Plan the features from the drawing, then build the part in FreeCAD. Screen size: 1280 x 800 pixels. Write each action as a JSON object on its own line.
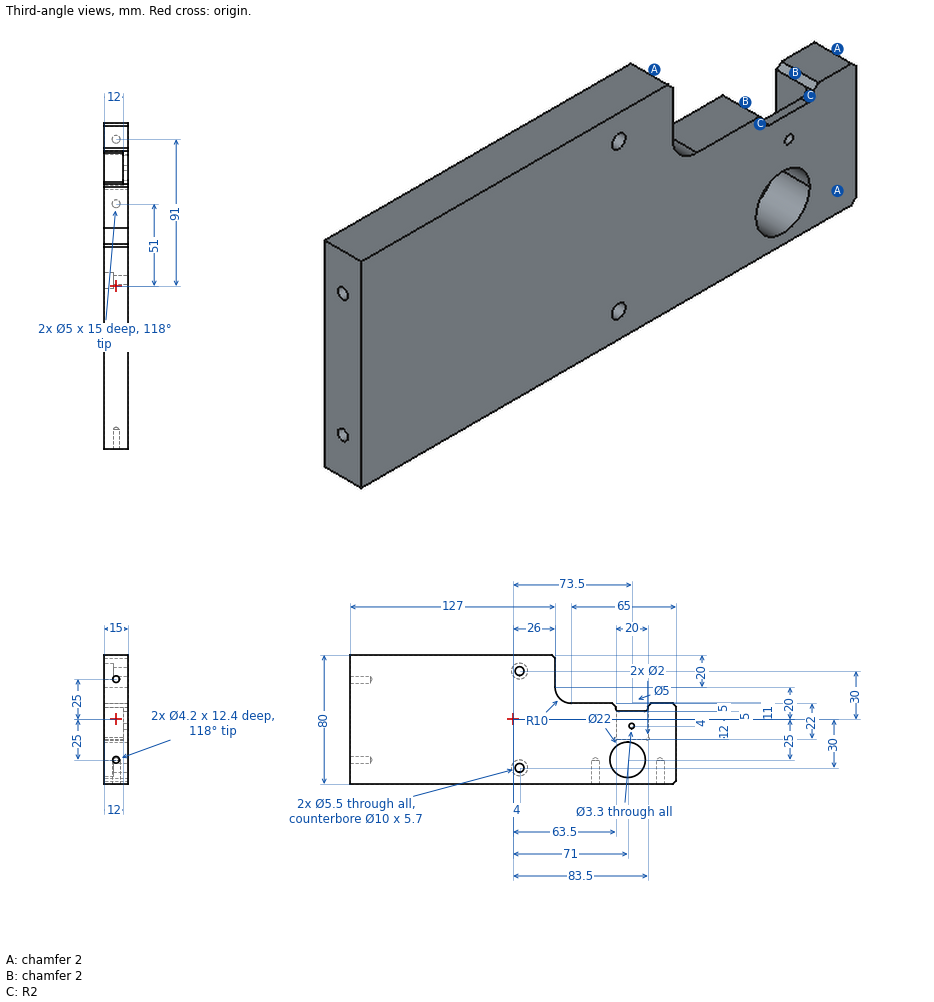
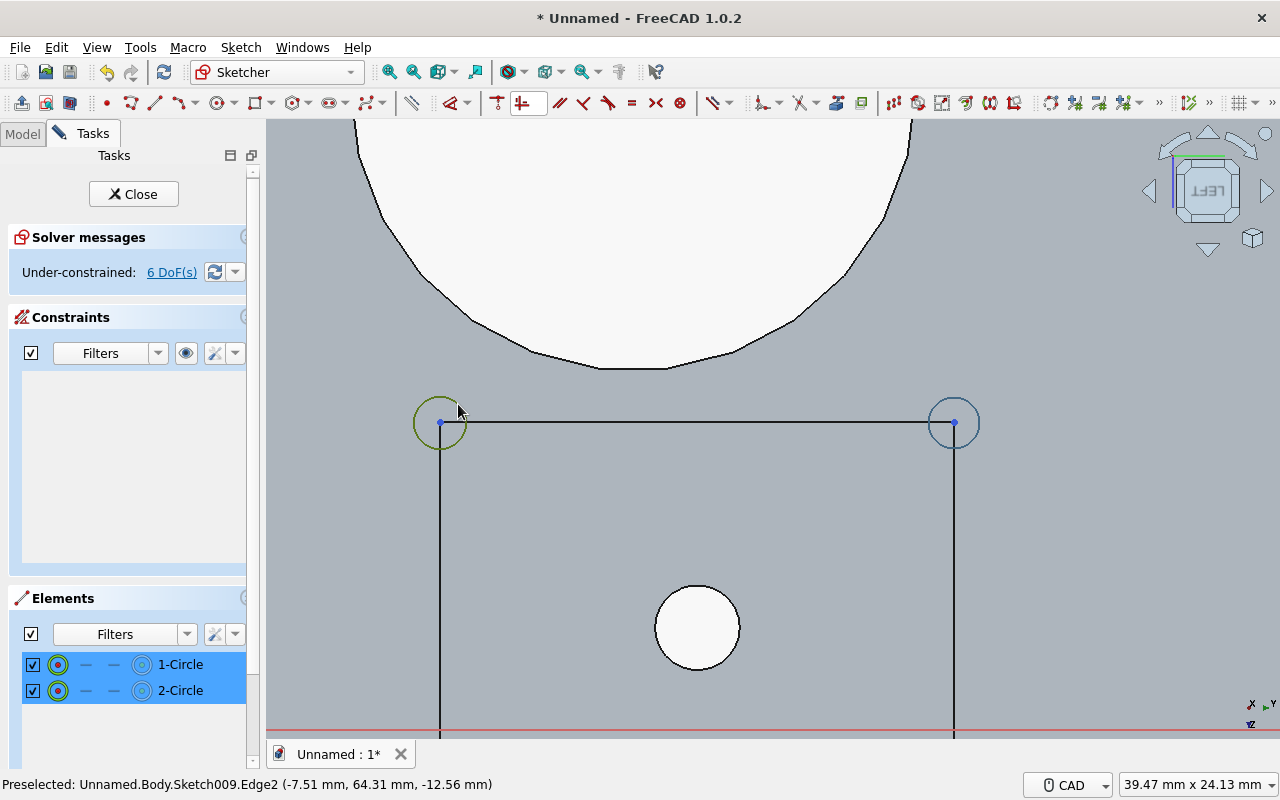
{"action": "left_click", "coordinate": [632, 104]}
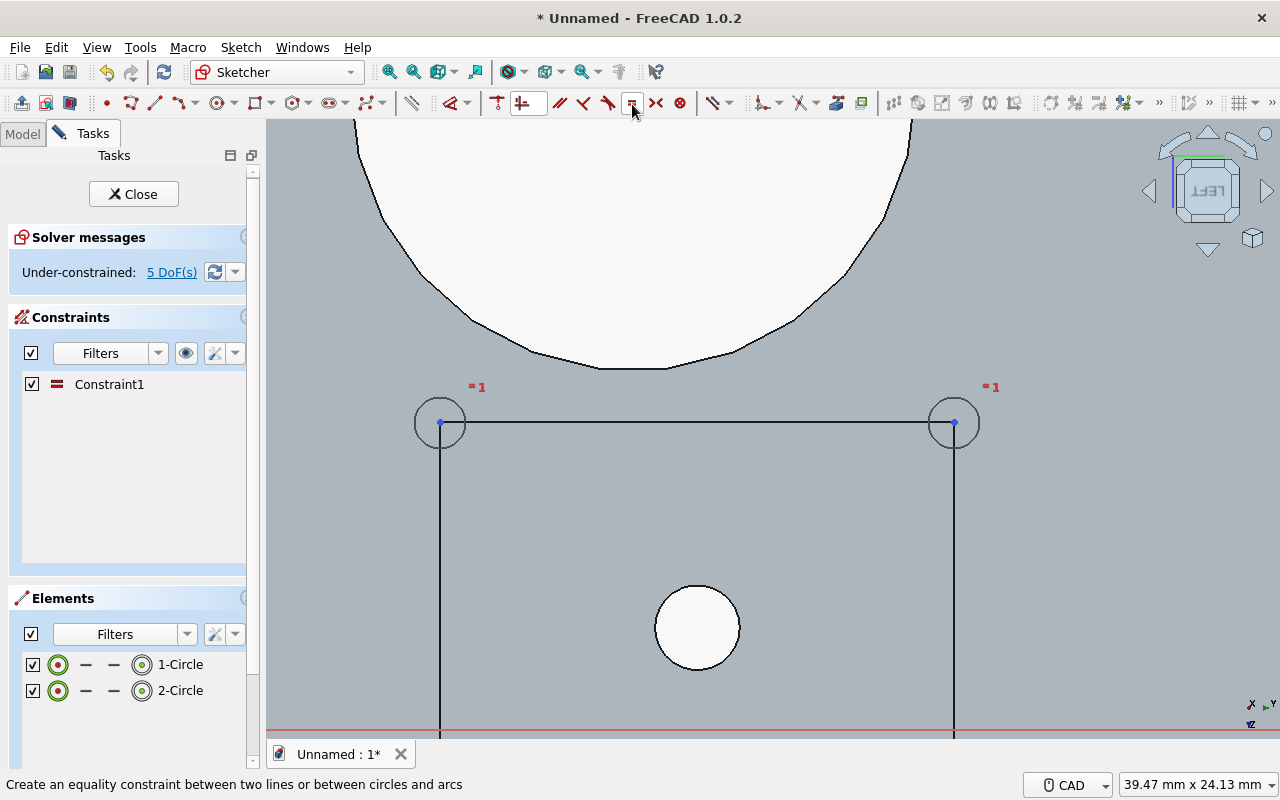
{"action": "left_click", "coordinate": [954, 423]}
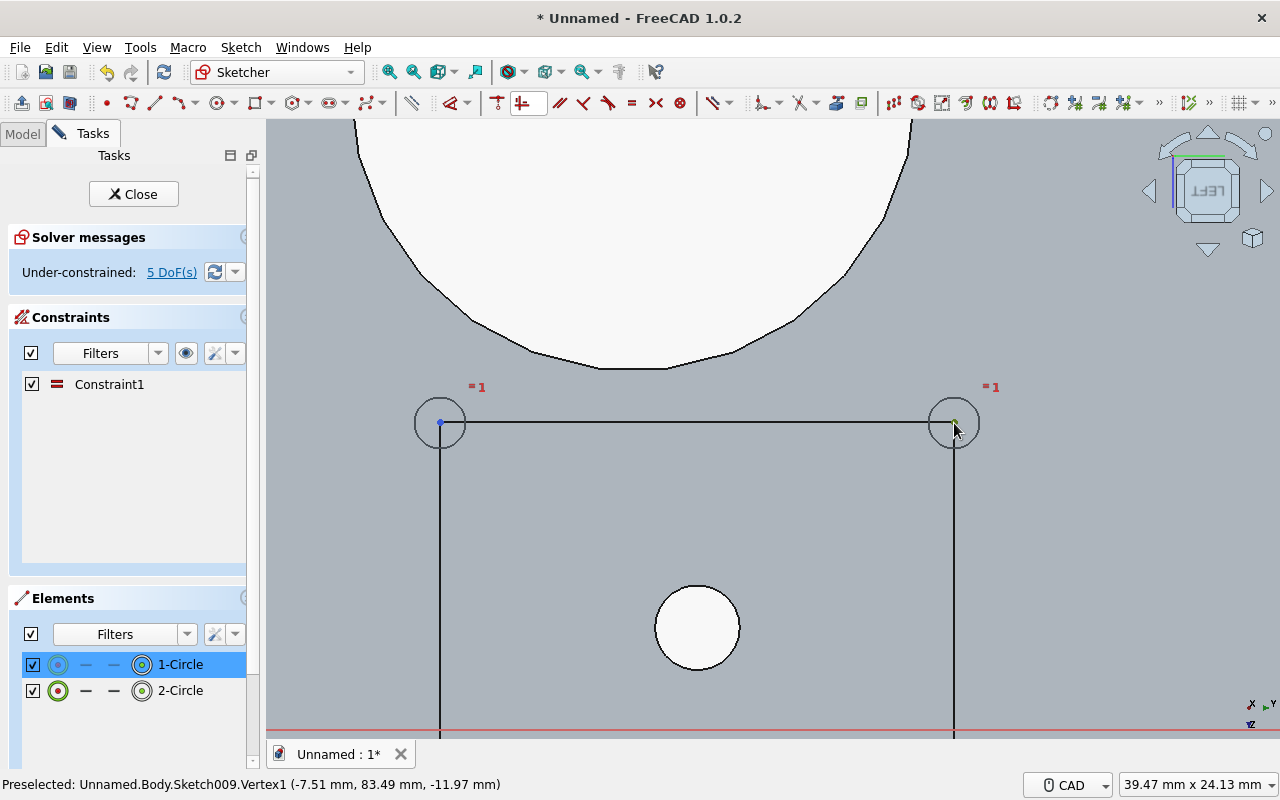
{"action": "left_click", "coordinate": [440, 423]}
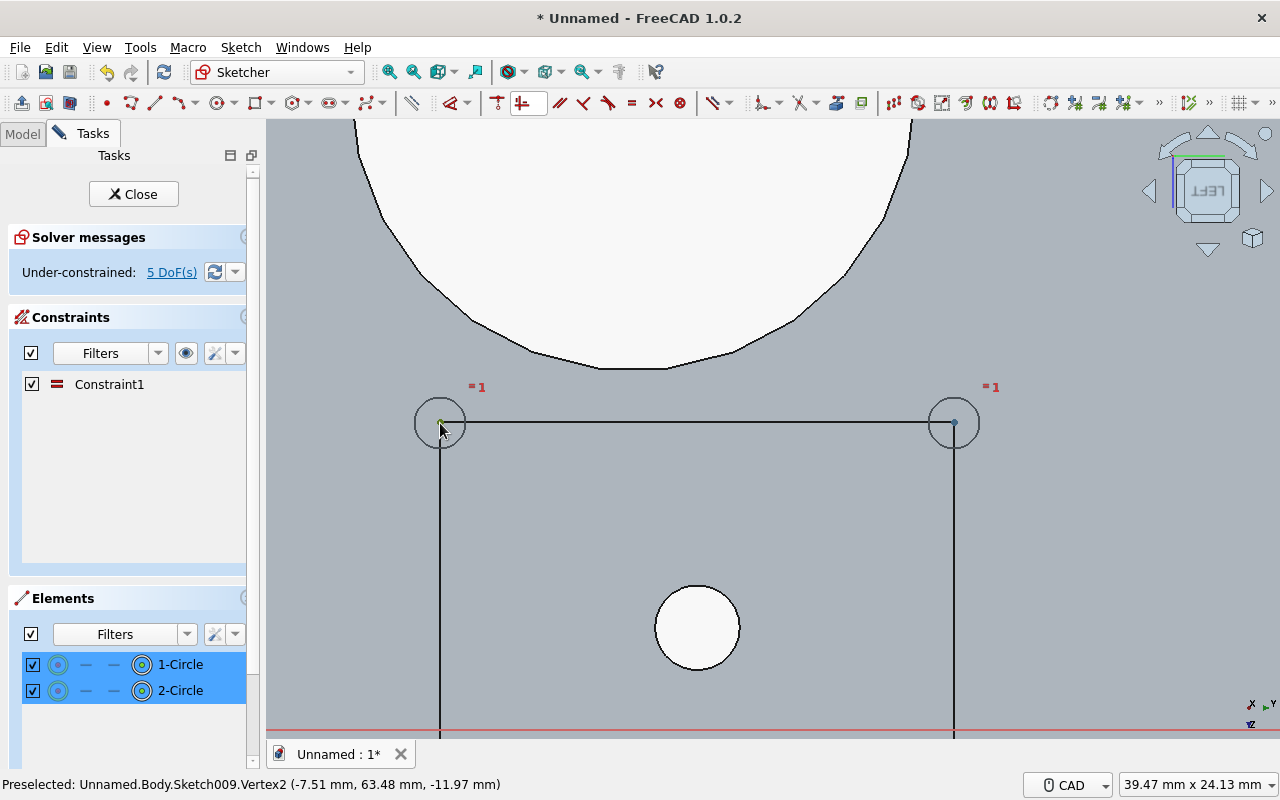
{"action": "left_click", "coordinate": [542, 104]}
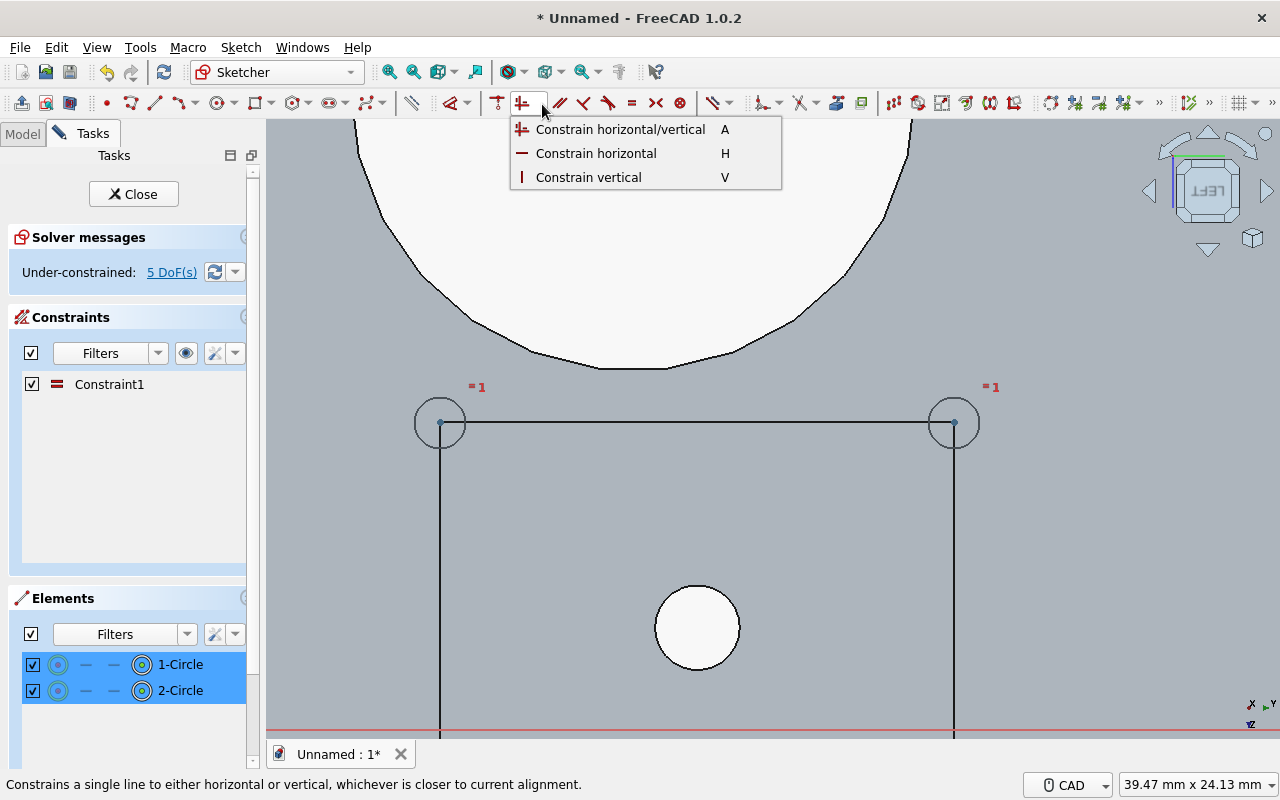
{"action": "left_click", "coordinate": [646, 153]}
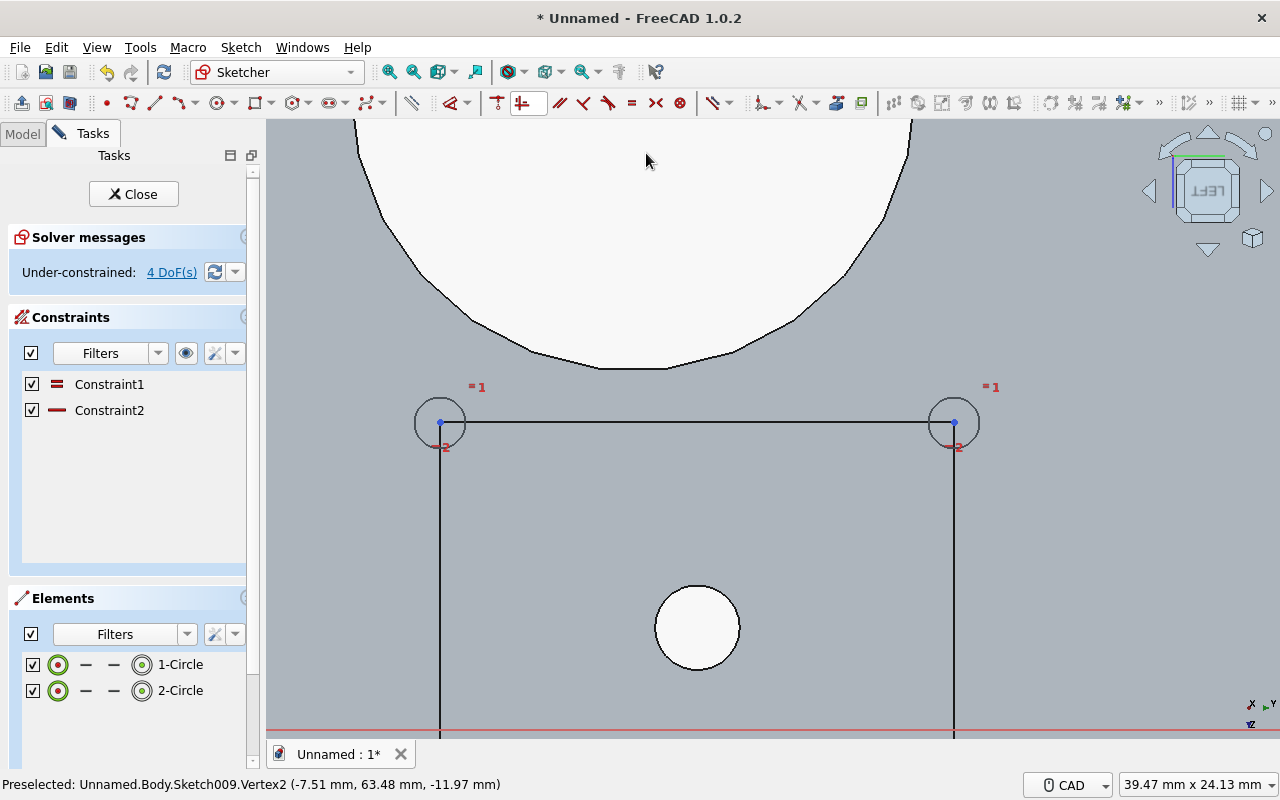
{"action": "left_click", "coordinate": [450, 104]}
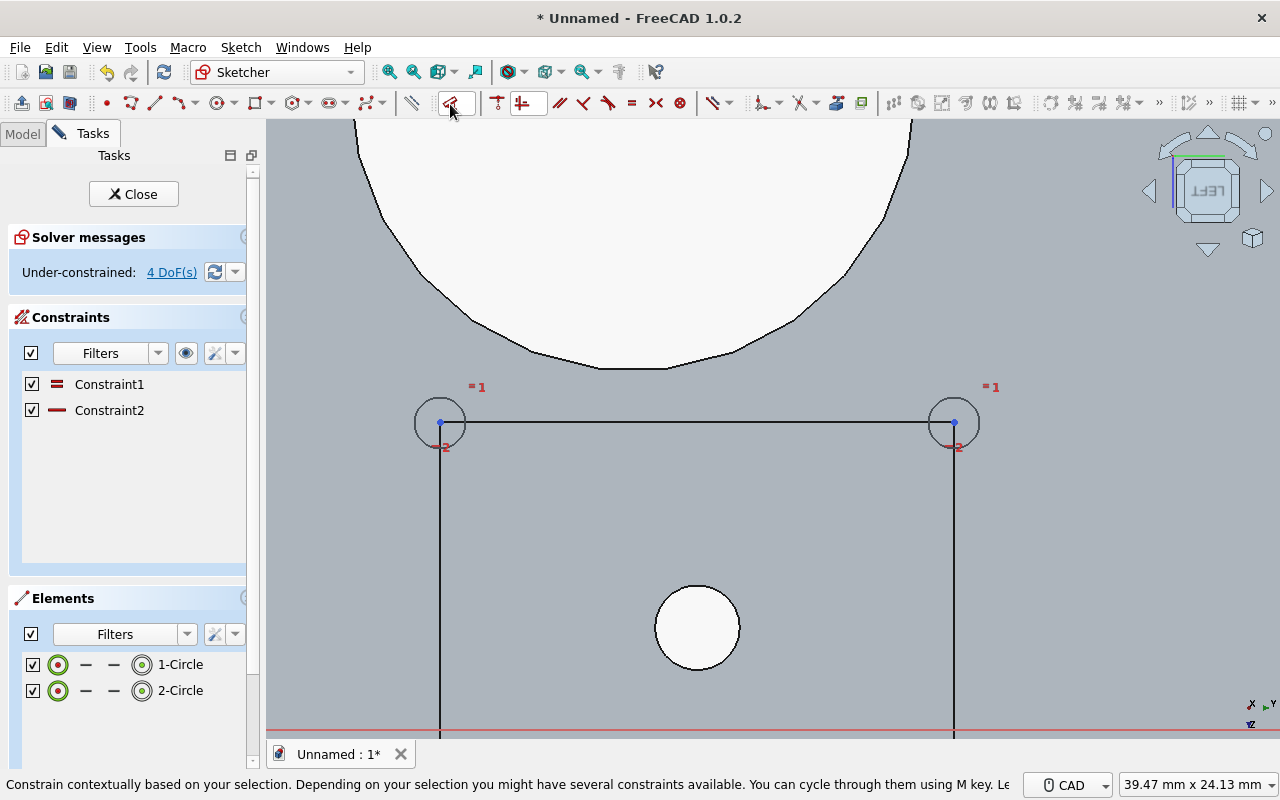
{"action": "left_click", "coordinate": [972, 405]}
{"action": "left_click", "coordinate": [995, 382]}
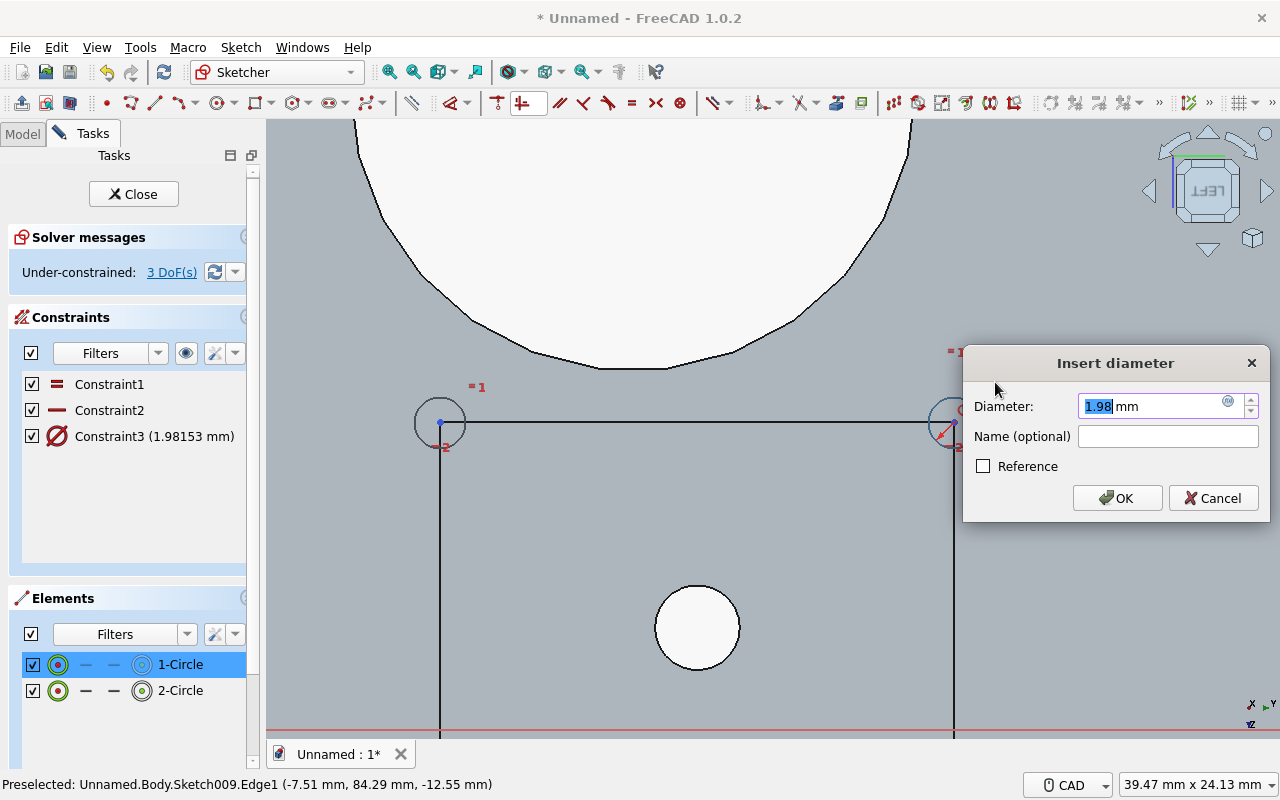
{"action": "type", "text": "2"}
{"action": "key", "text": "Return"}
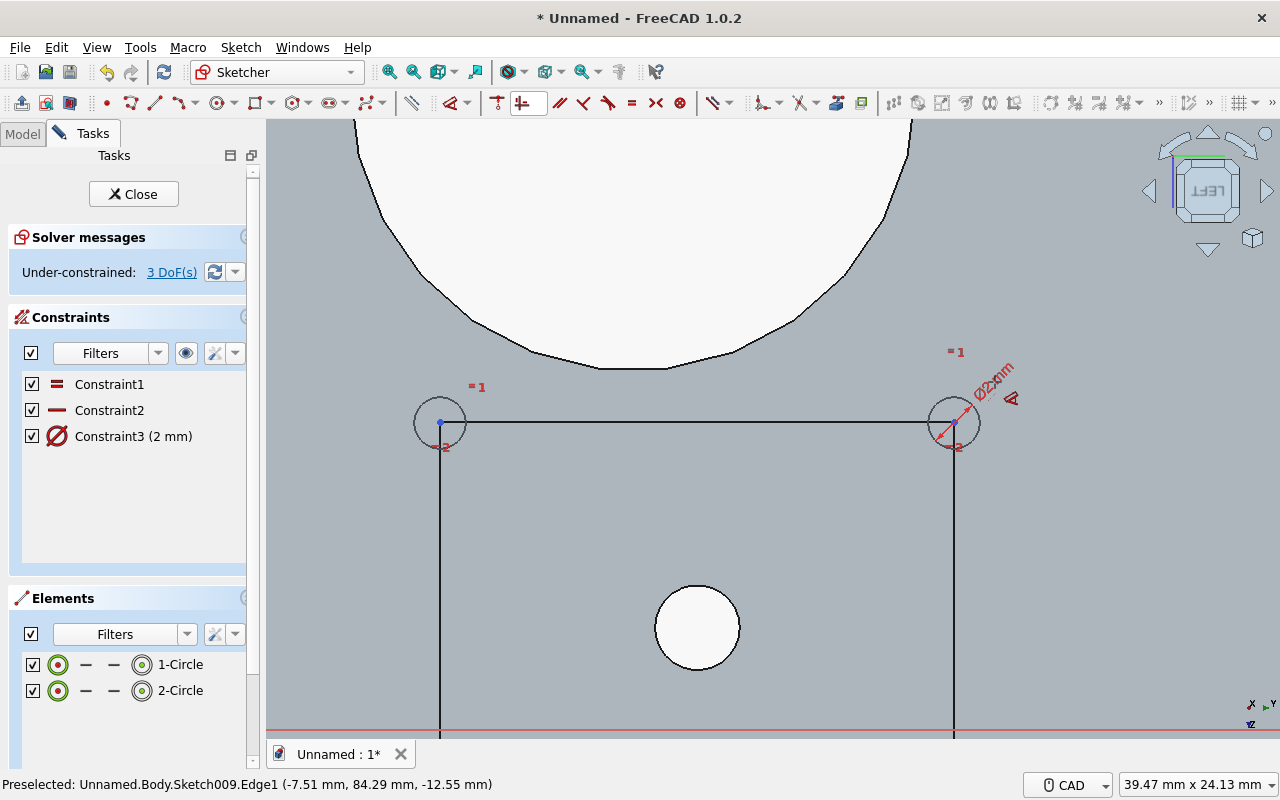
{"action": "left_click", "coordinate": [954, 423]}
{"action": "left_click", "coordinate": [988, 567]}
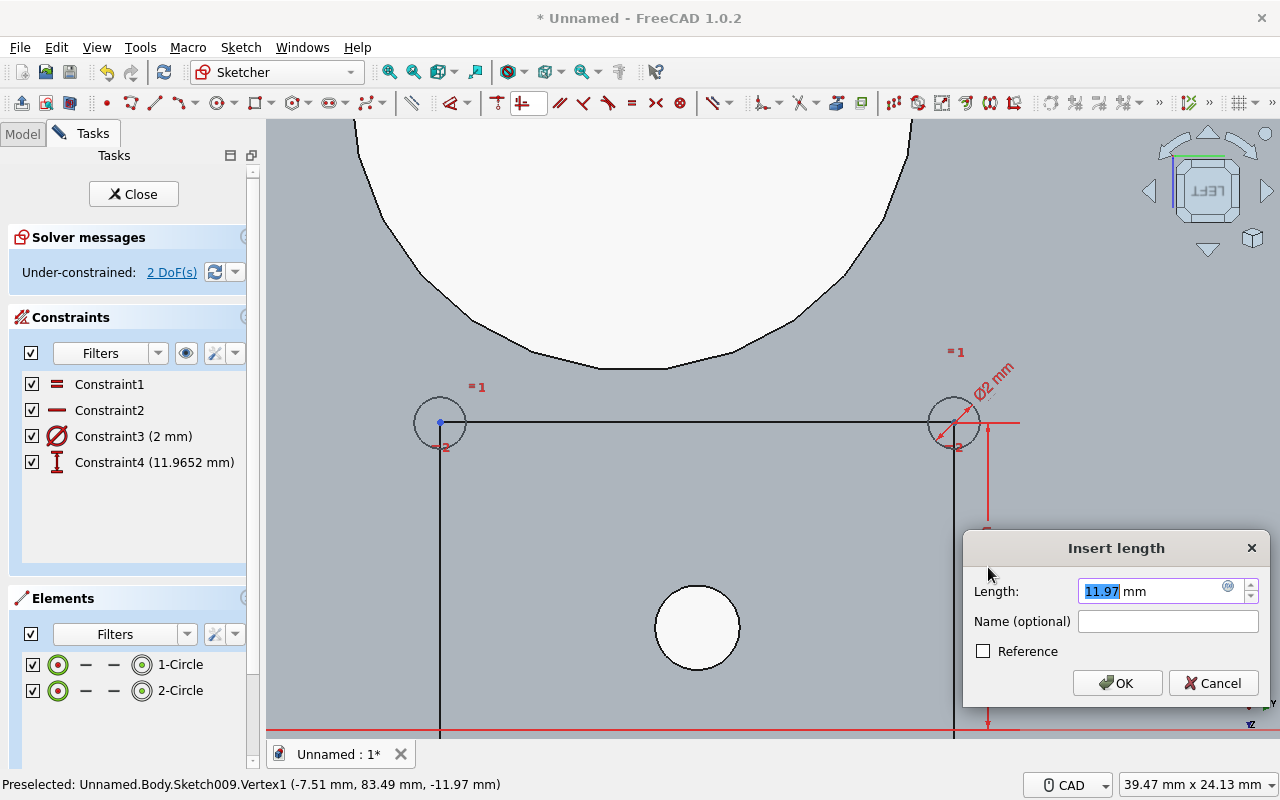
{"action": "type", "text": "12"}
{"action": "key", "text": "Return"}